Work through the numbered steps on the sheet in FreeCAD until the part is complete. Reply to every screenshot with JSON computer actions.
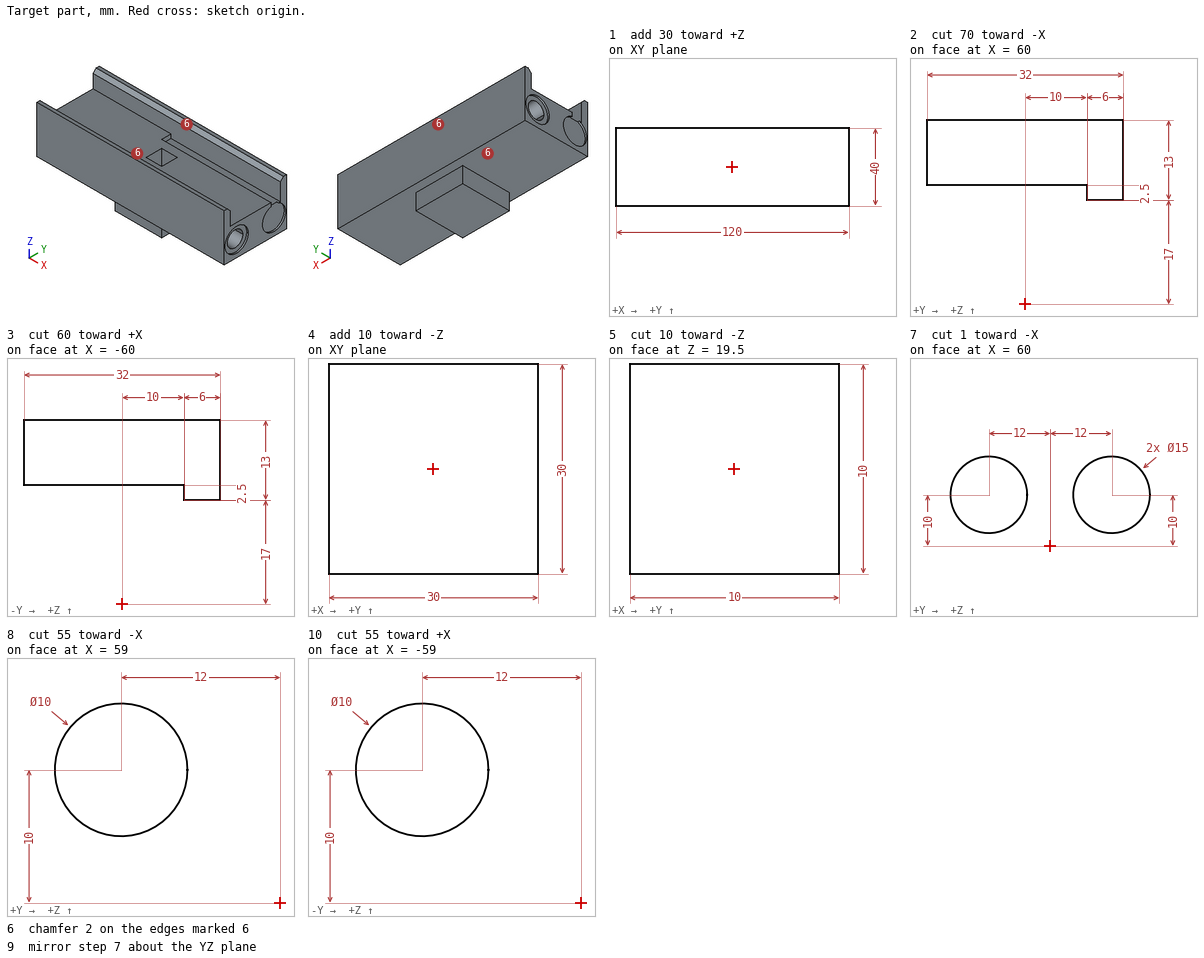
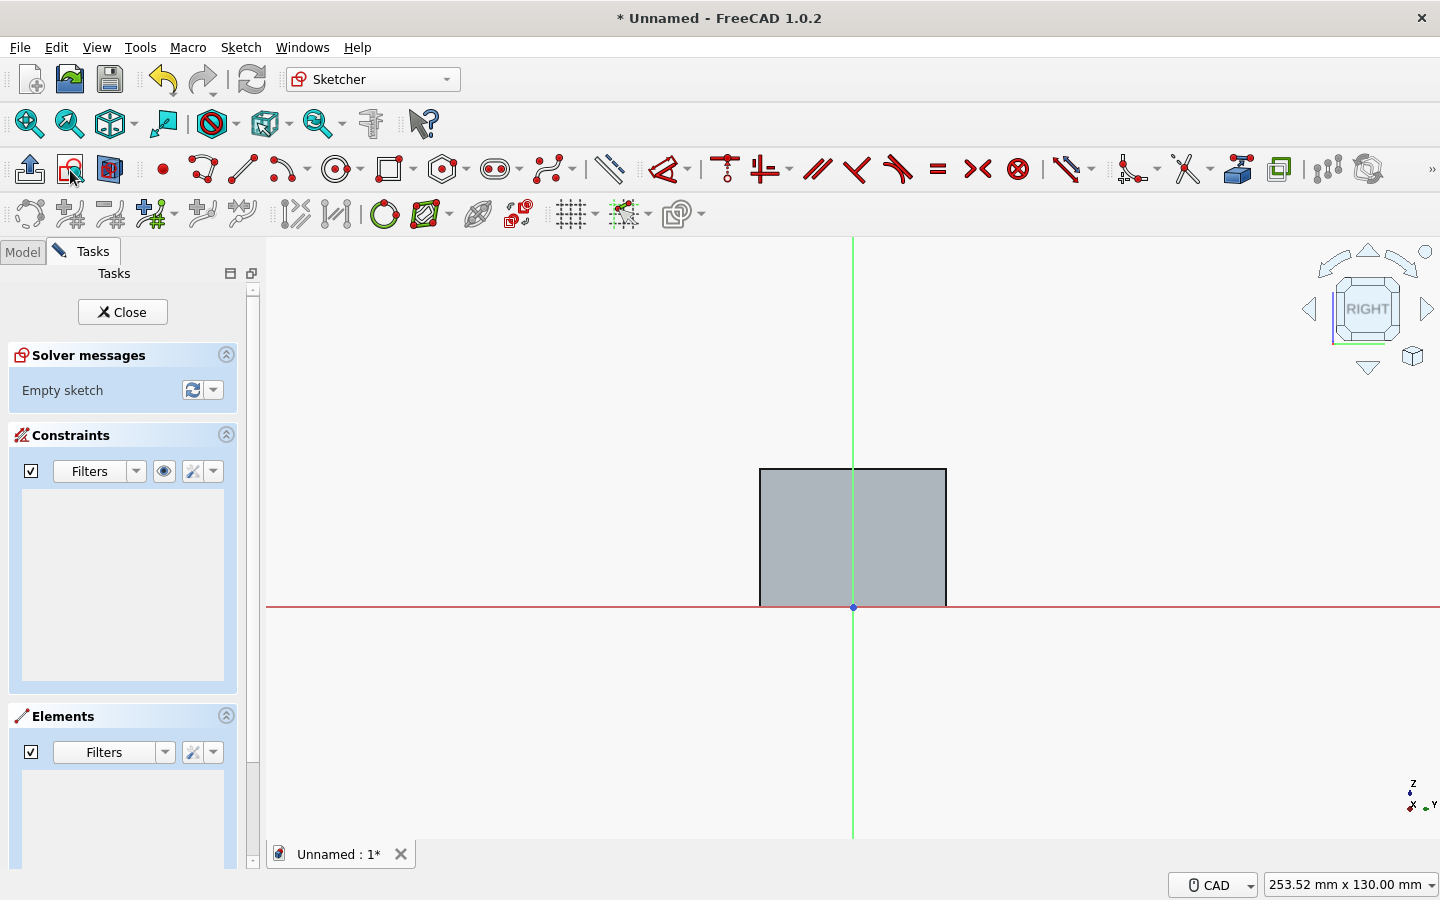
{"action": "scroll", "coordinate": [893, 538], "scroll_direction": "up", "scroll_amount": 5}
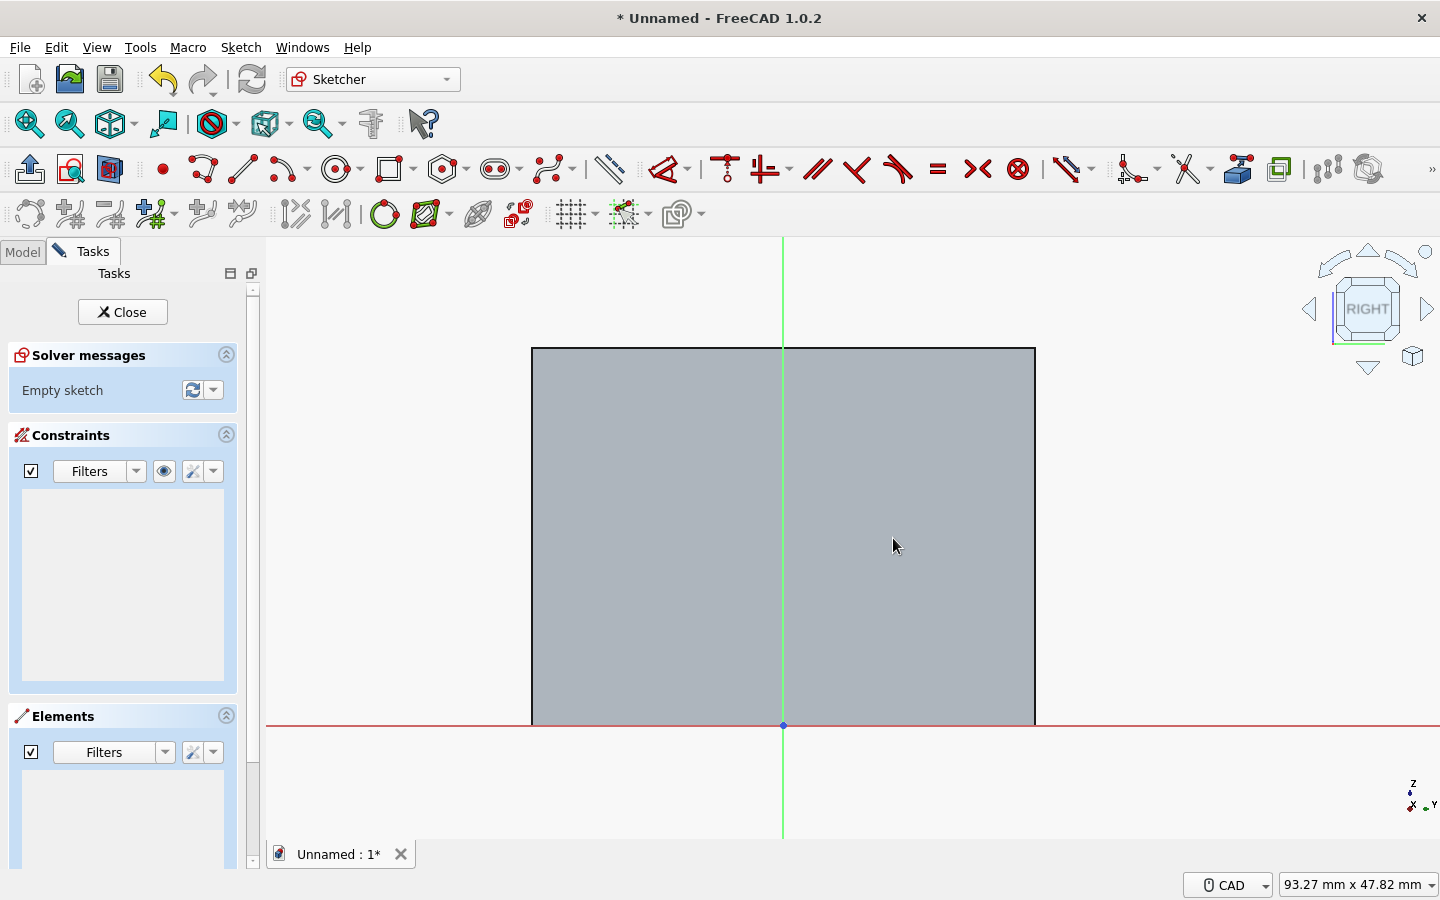
{"action": "key", "text": "g m"}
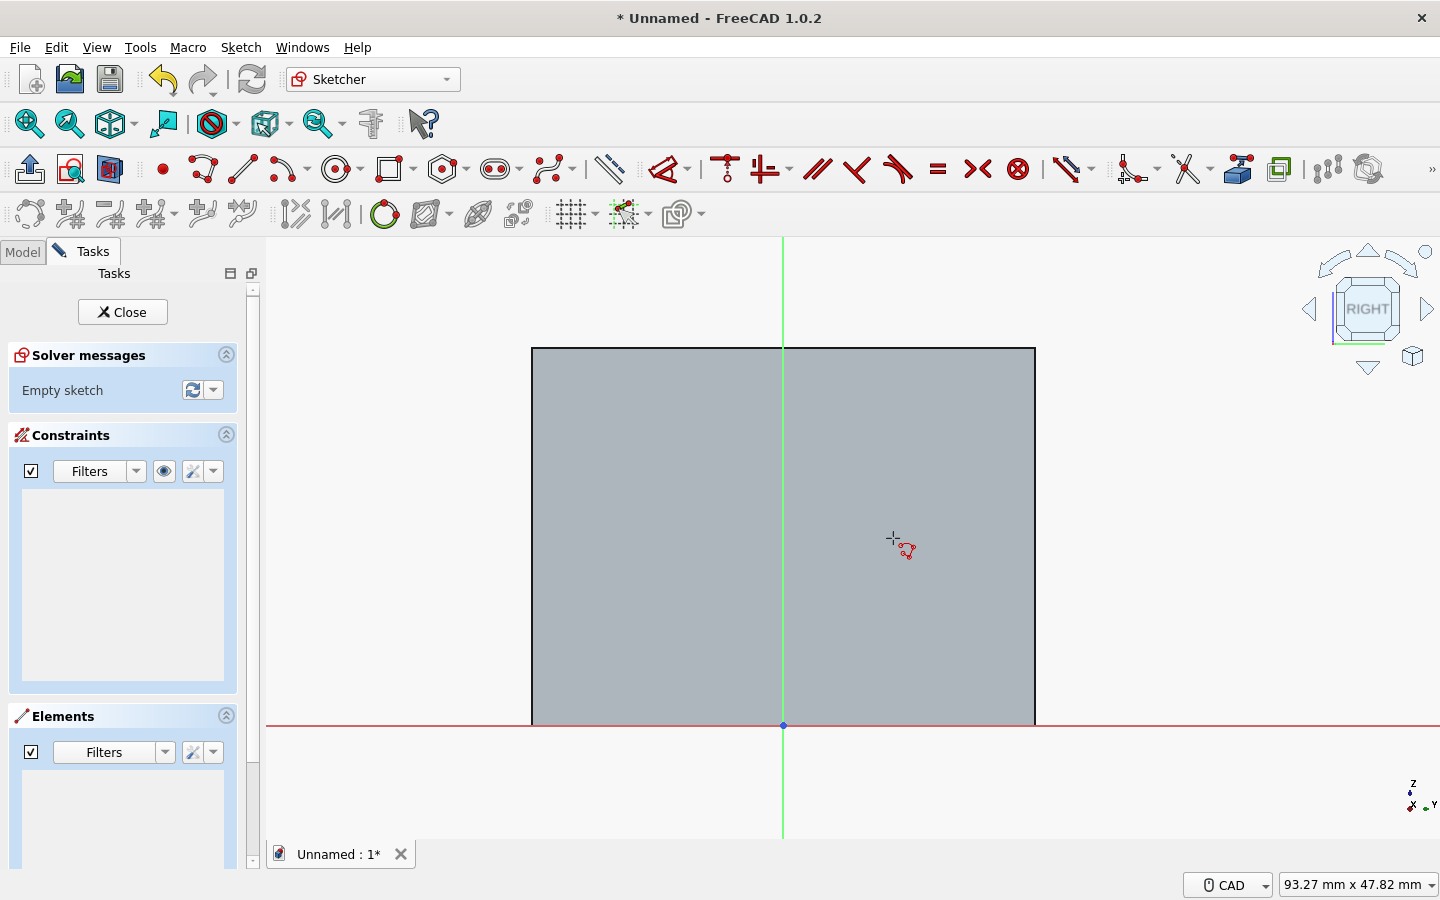
{"action": "left_click", "coordinate": [909, 512]}
{"action": "left_click", "coordinate": [985, 512]}
{"action": "left_click", "coordinate": [985, 348]}
{"action": "left_click", "coordinate": [582, 348]}
{"action": "left_click", "coordinate": [582, 480]}
{"action": "left_click", "coordinate": [909, 480]}
{"action": "left_click", "coordinate": [909, 513]}
{"action": "key", "text": "Escape"}
{"action": "key", "text": "Escape"}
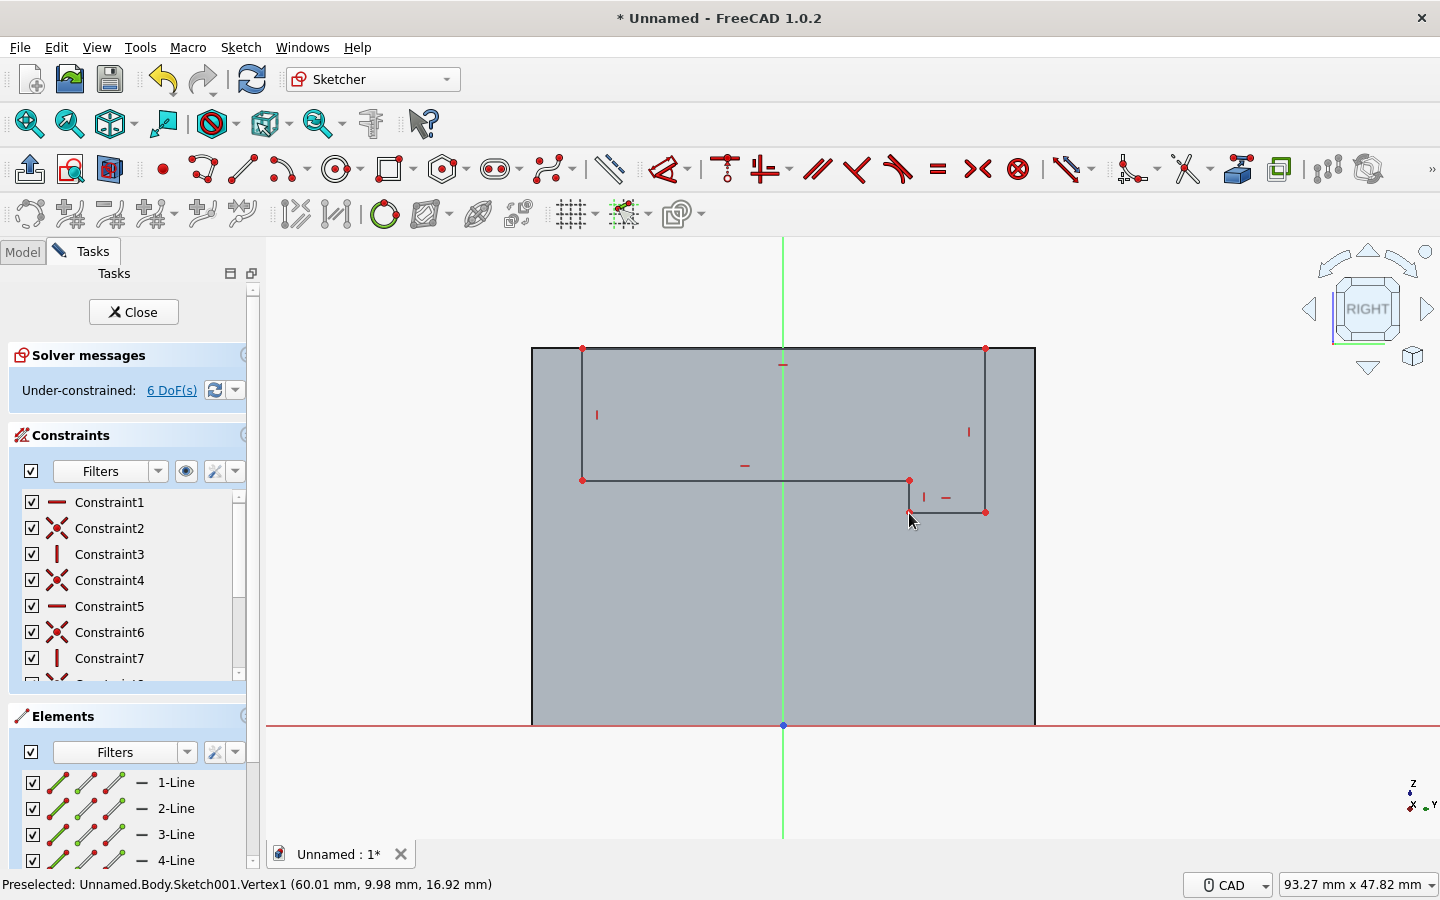
{"action": "key", "text": "d"}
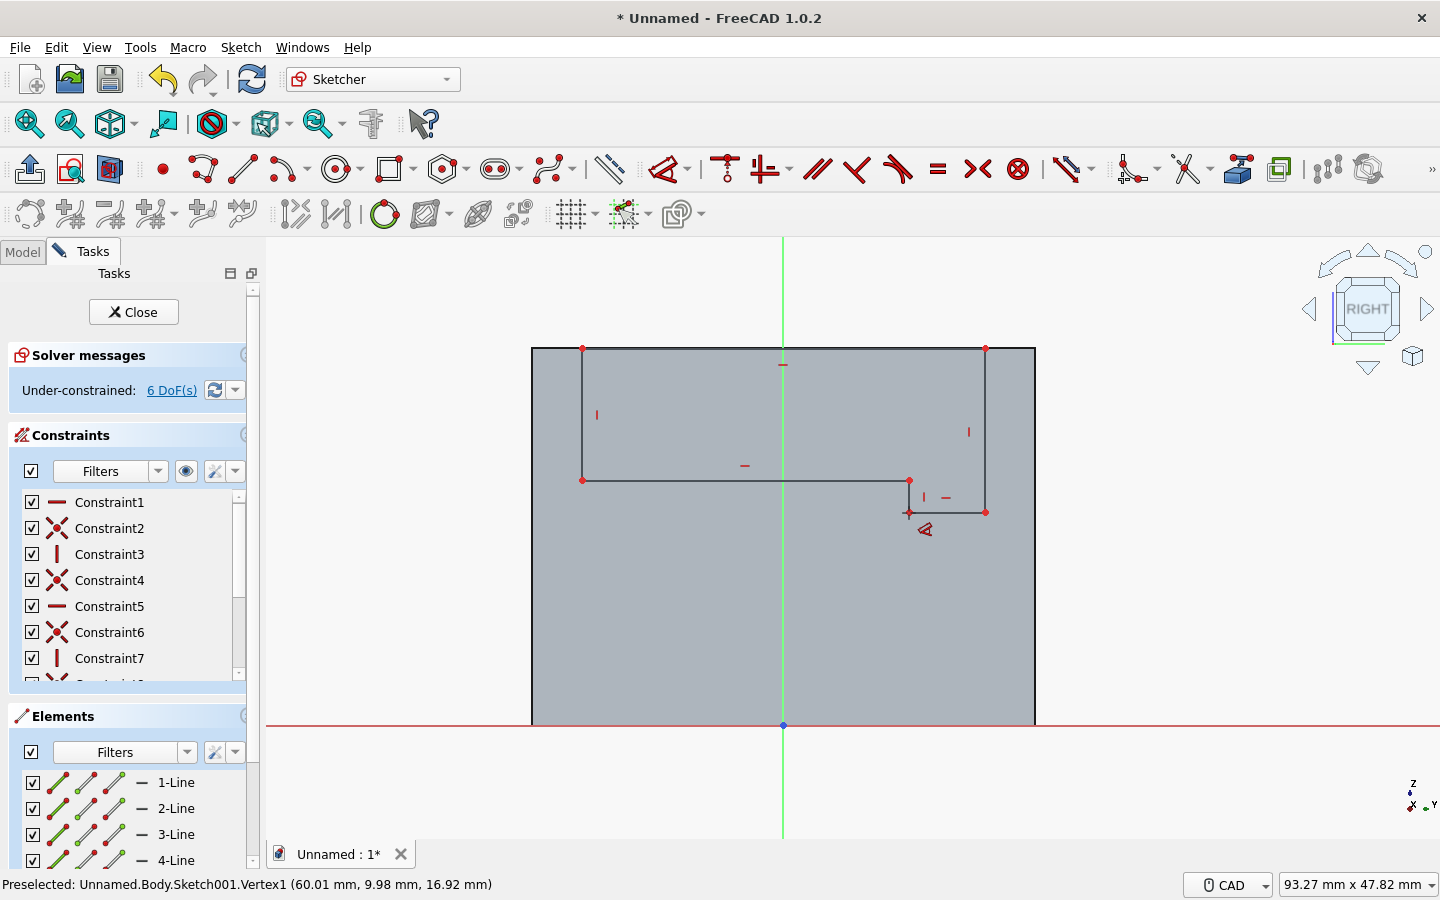
{"action": "left_click", "coordinate": [932, 513]}
{"action": "left_click", "coordinate": [947, 479]}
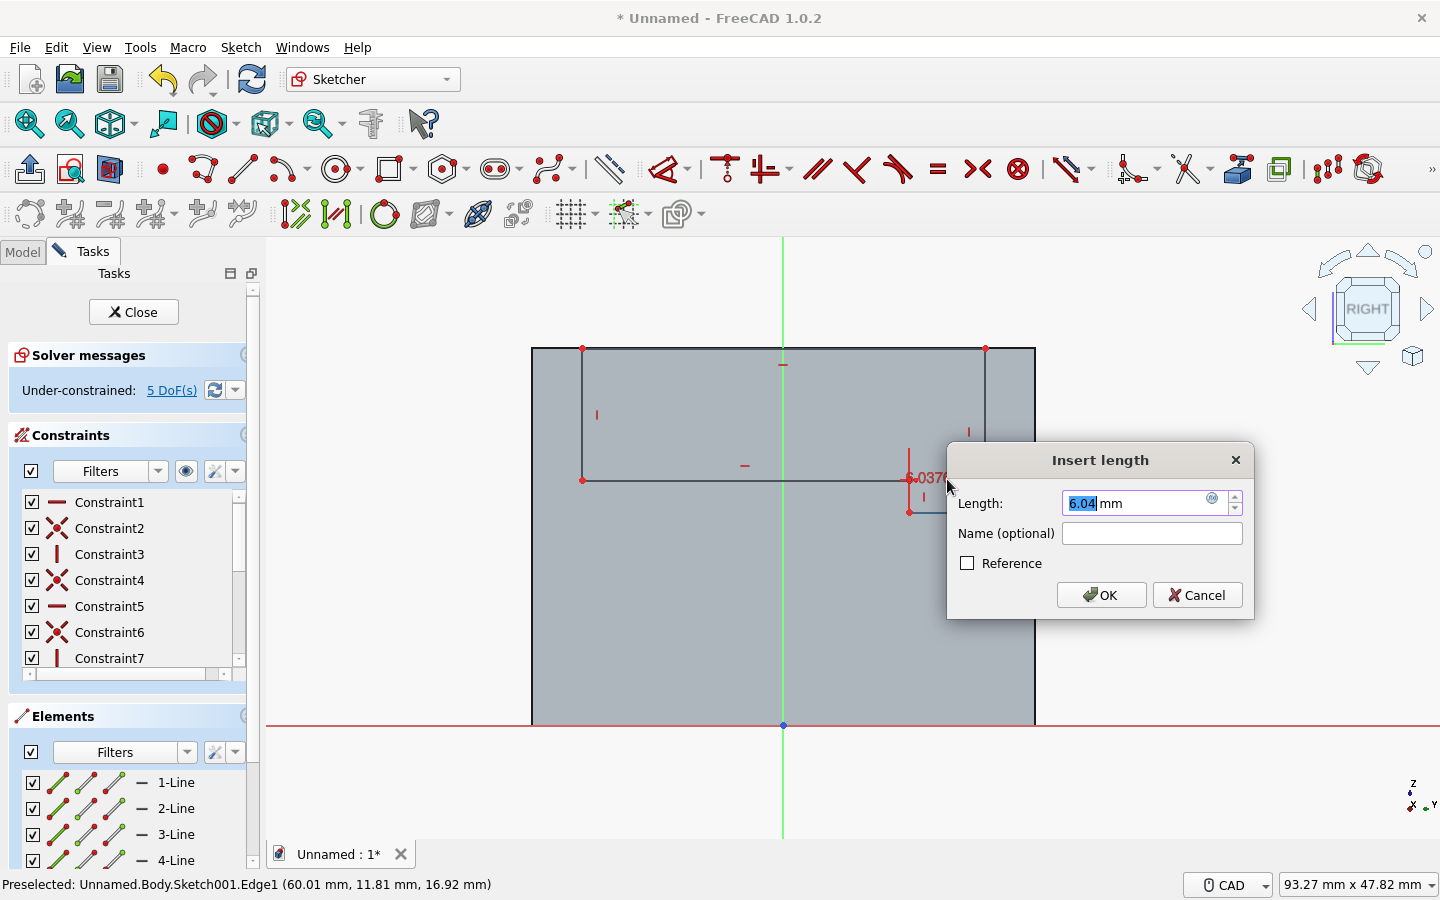
{"action": "type", "text": "6"}
{"action": "key", "text": "Return"}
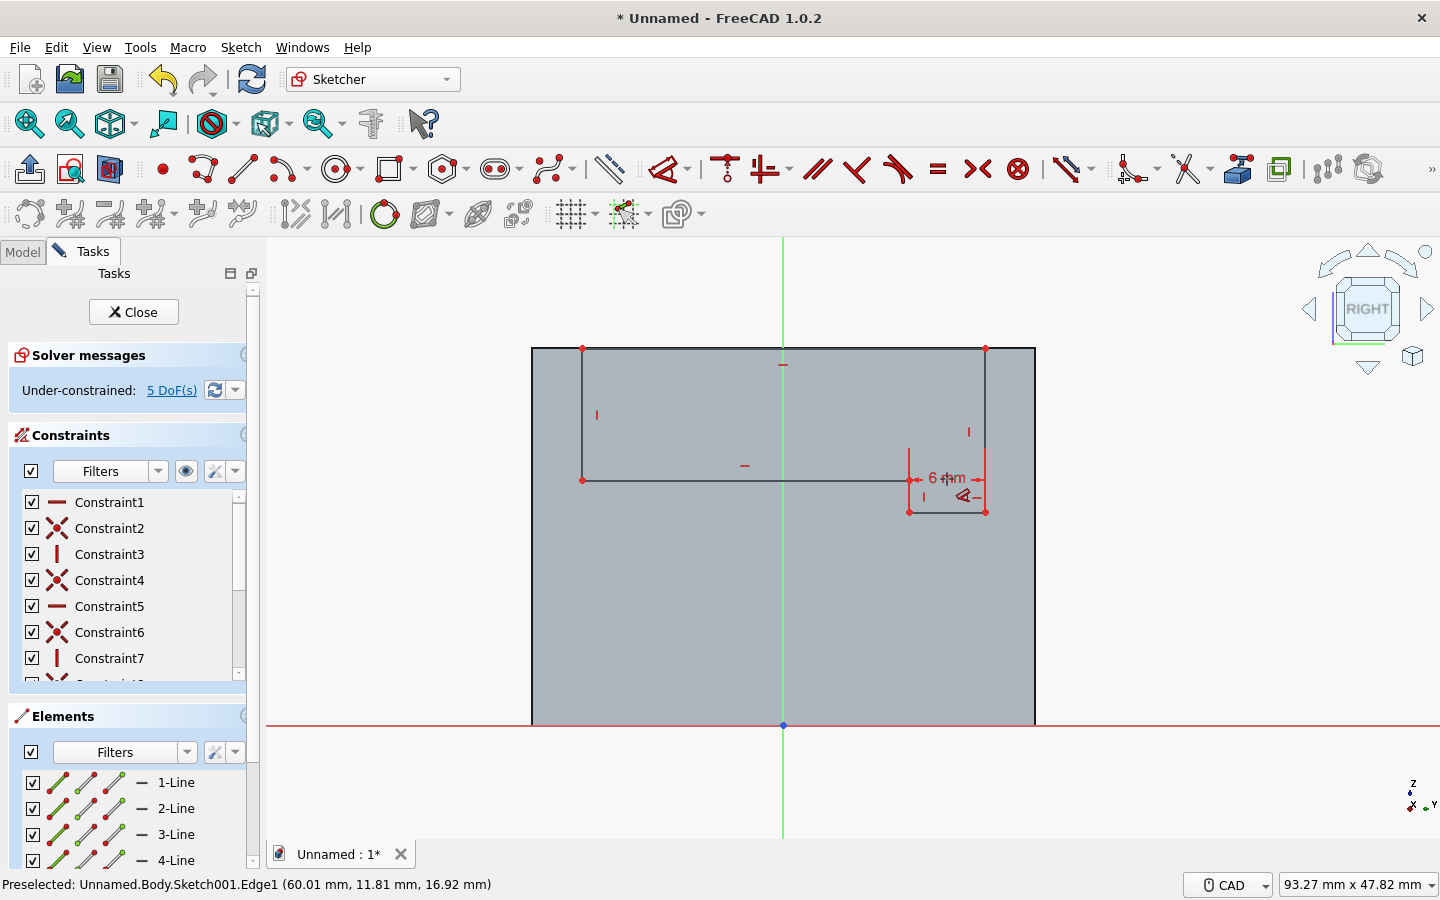
{"action": "left_click", "coordinate": [985, 464]}
{"action": "left_click", "coordinate": [1019, 431]}